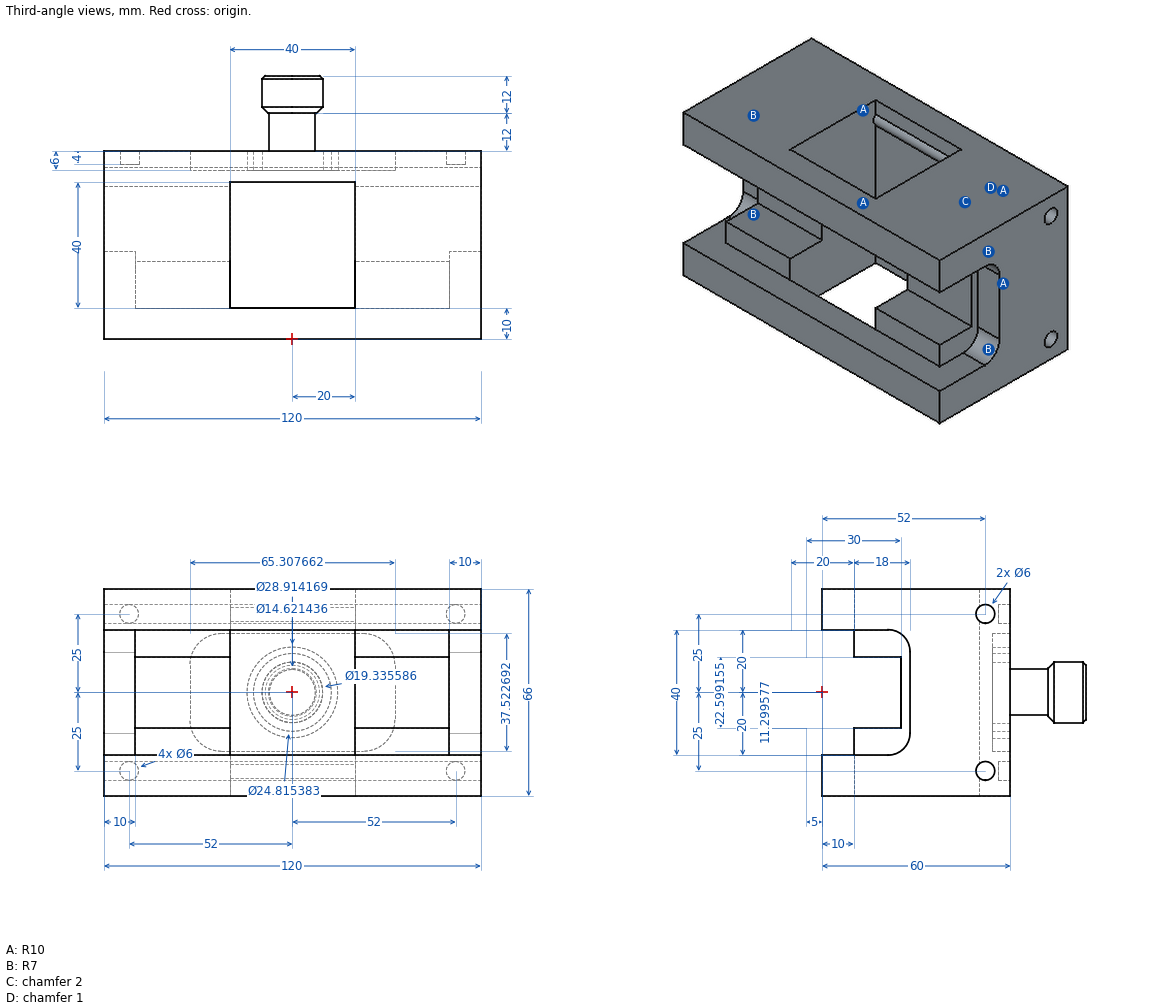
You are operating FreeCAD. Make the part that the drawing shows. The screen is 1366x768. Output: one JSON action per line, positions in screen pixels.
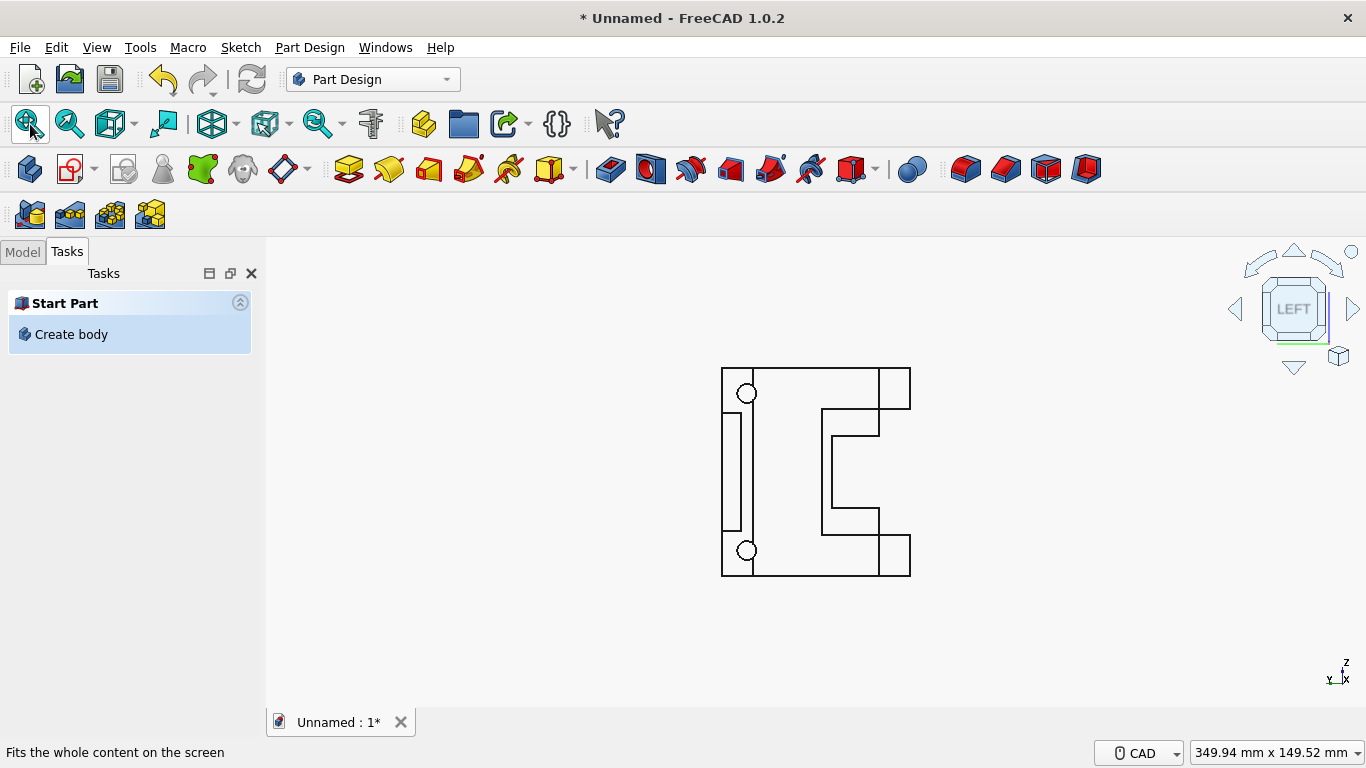
{"action": "key", "text": "0"}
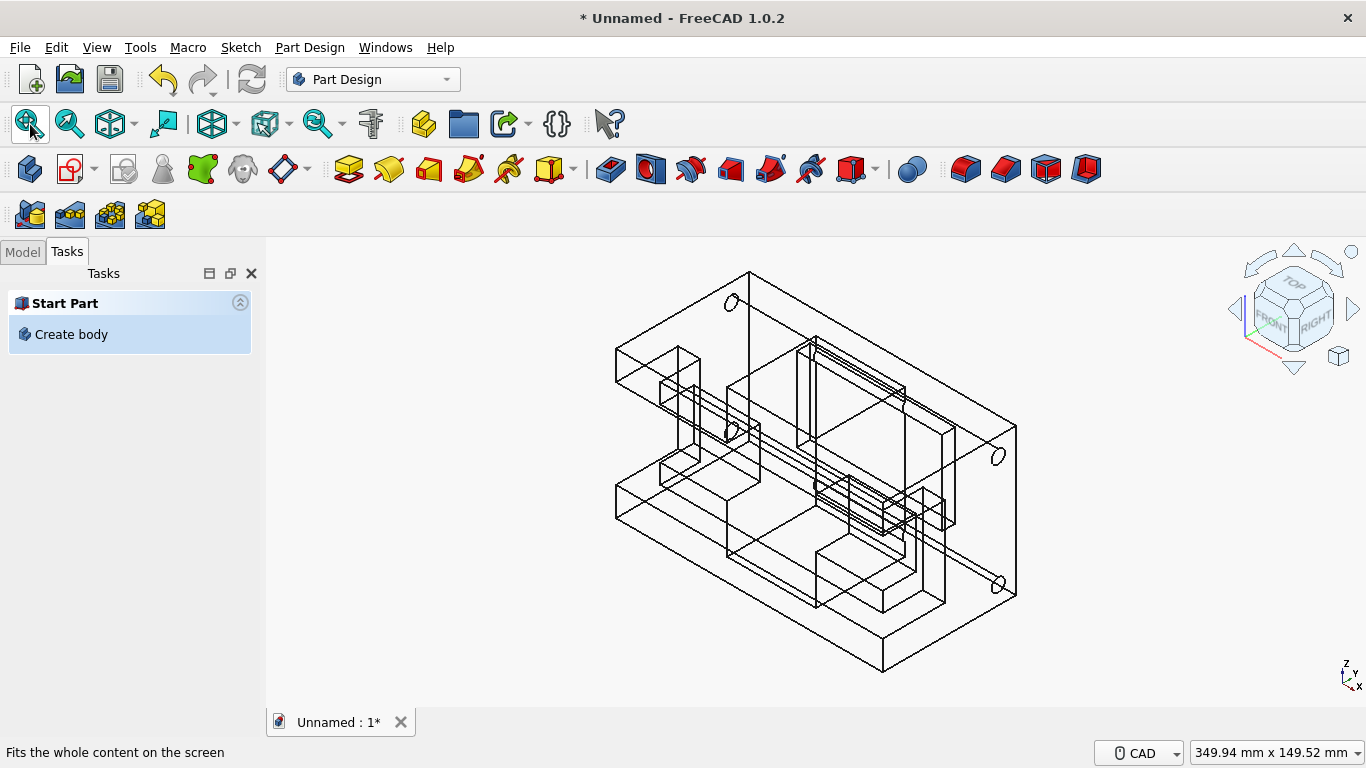
{"action": "left_click", "coordinate": [951, 525]}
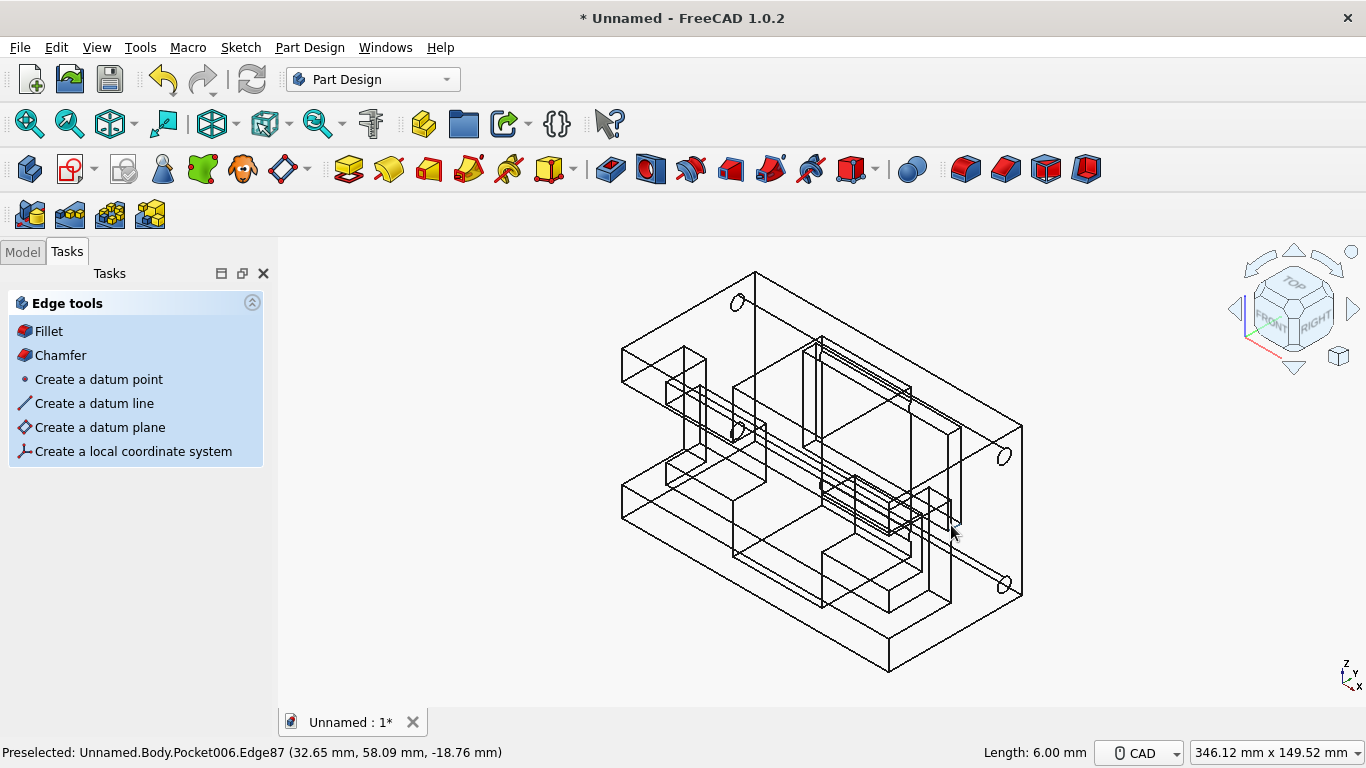
{"action": "left_click", "coordinate": [955, 430], "text": "ctrl"}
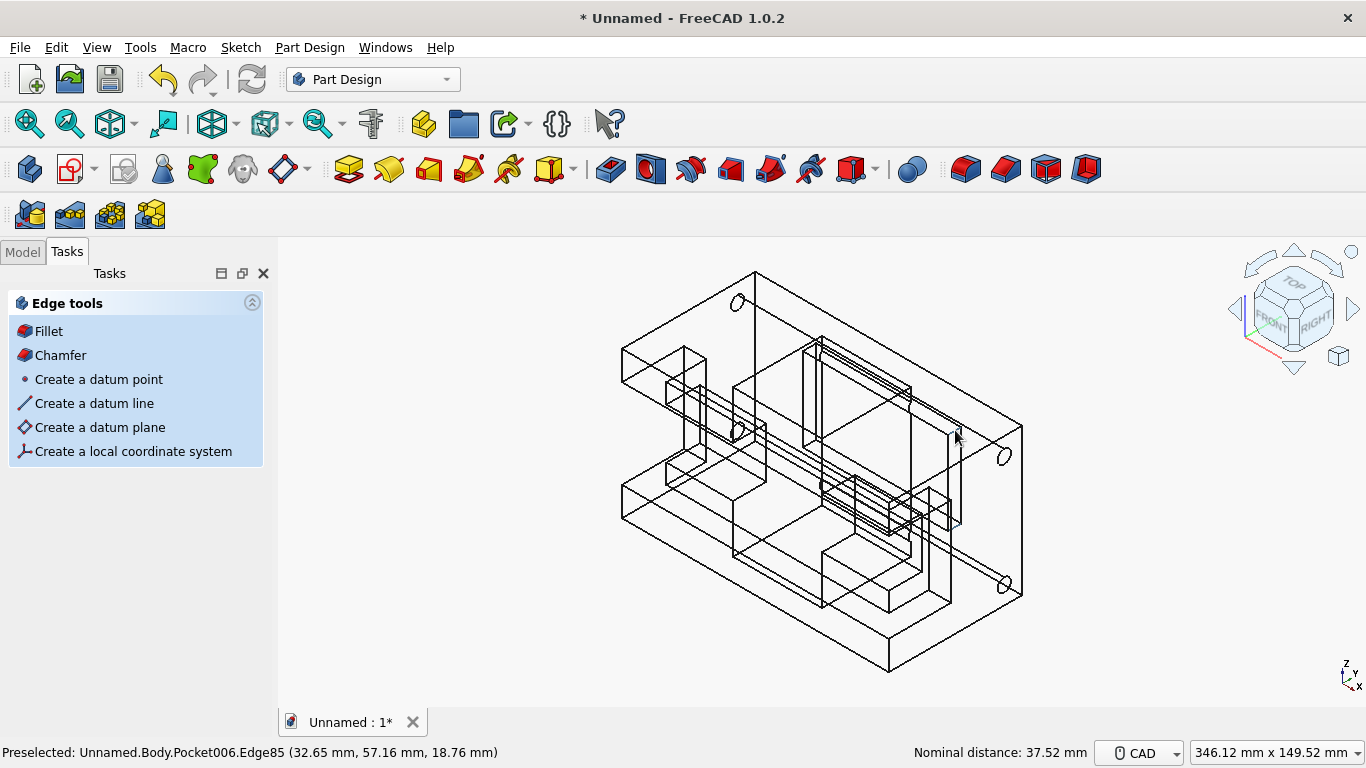
{"action": "left_click", "coordinate": [811, 442], "text": "ctrl"}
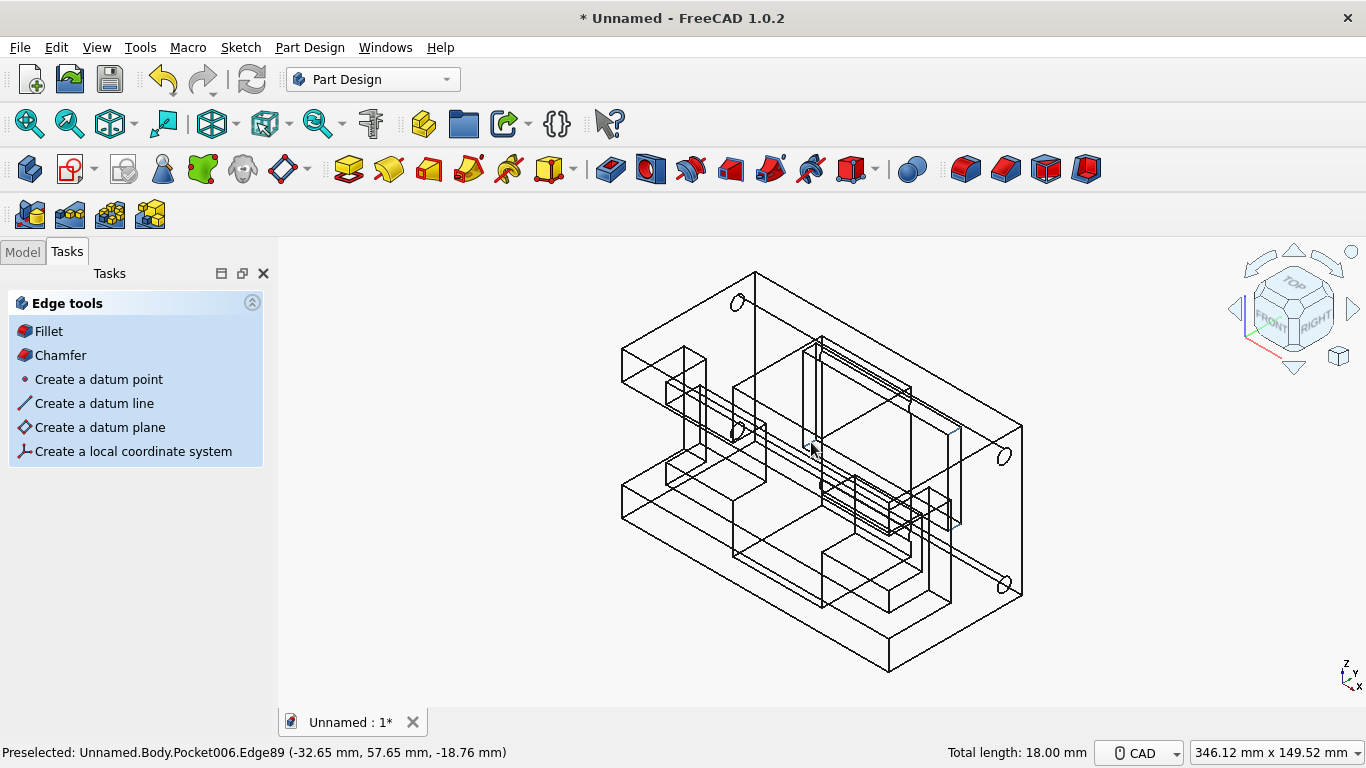
{"action": "scroll", "coordinate": [809, 346], "scroll_direction": "up", "scroll_amount": 4}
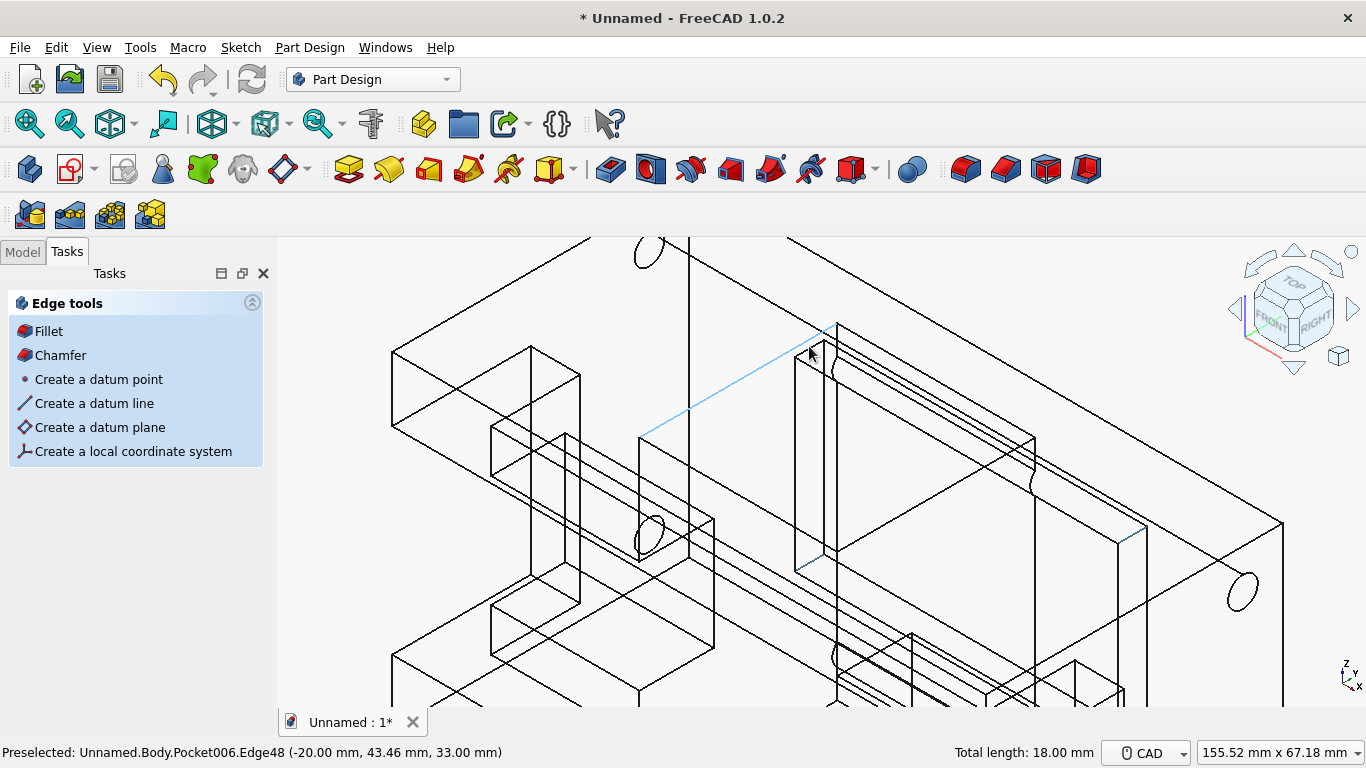
{"action": "left_click", "coordinate": [809, 348], "text": "ctrl"}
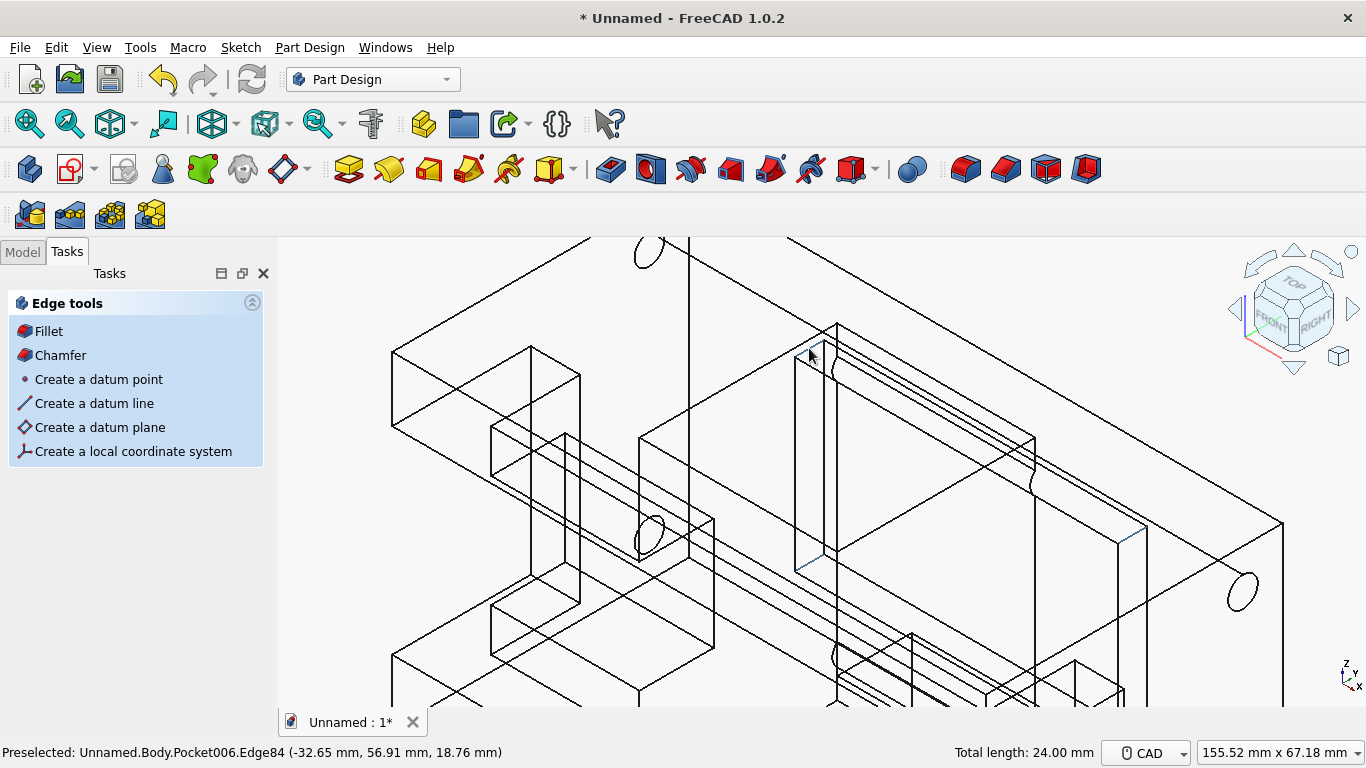
{"action": "key", "text": "v 1"}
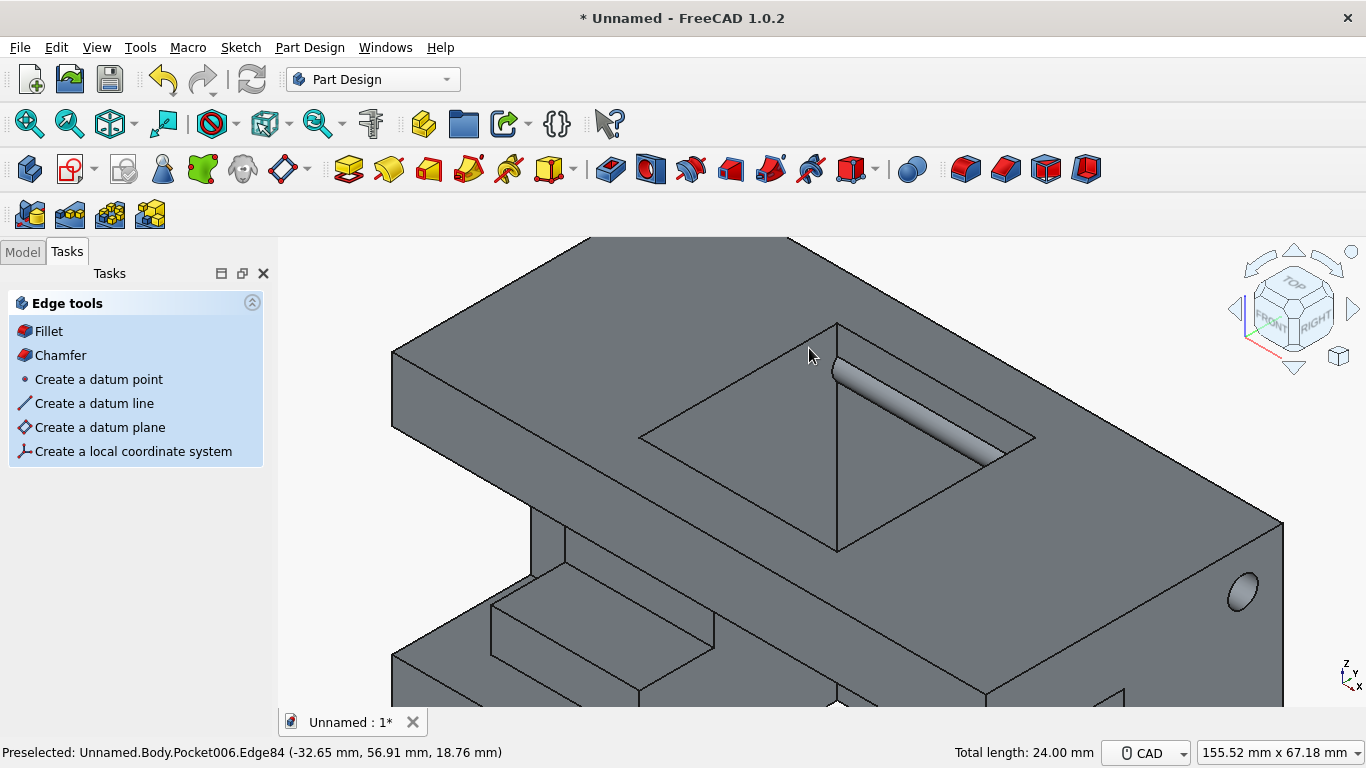
{"action": "left_click", "coordinate": [966, 170]}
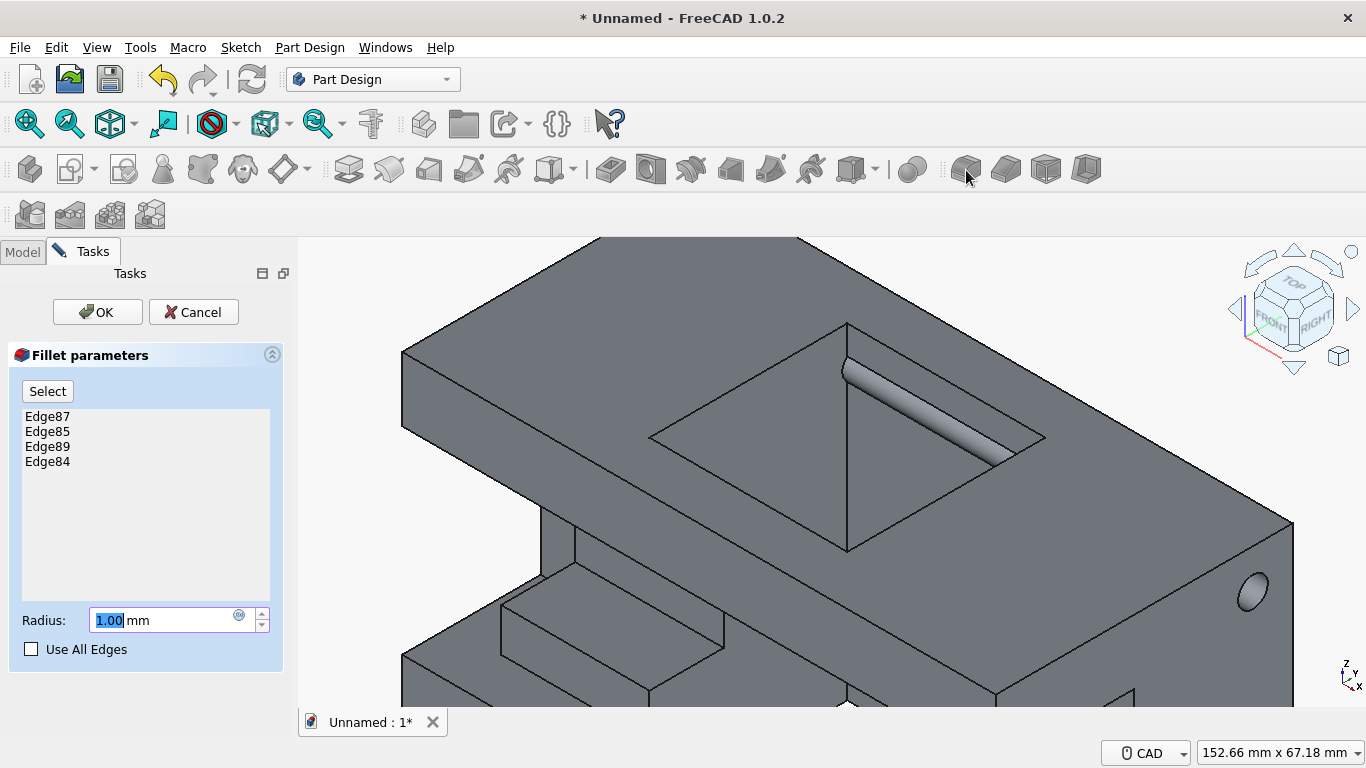
{"action": "type", "text": "10"}
{"action": "key", "text": "Tab"}